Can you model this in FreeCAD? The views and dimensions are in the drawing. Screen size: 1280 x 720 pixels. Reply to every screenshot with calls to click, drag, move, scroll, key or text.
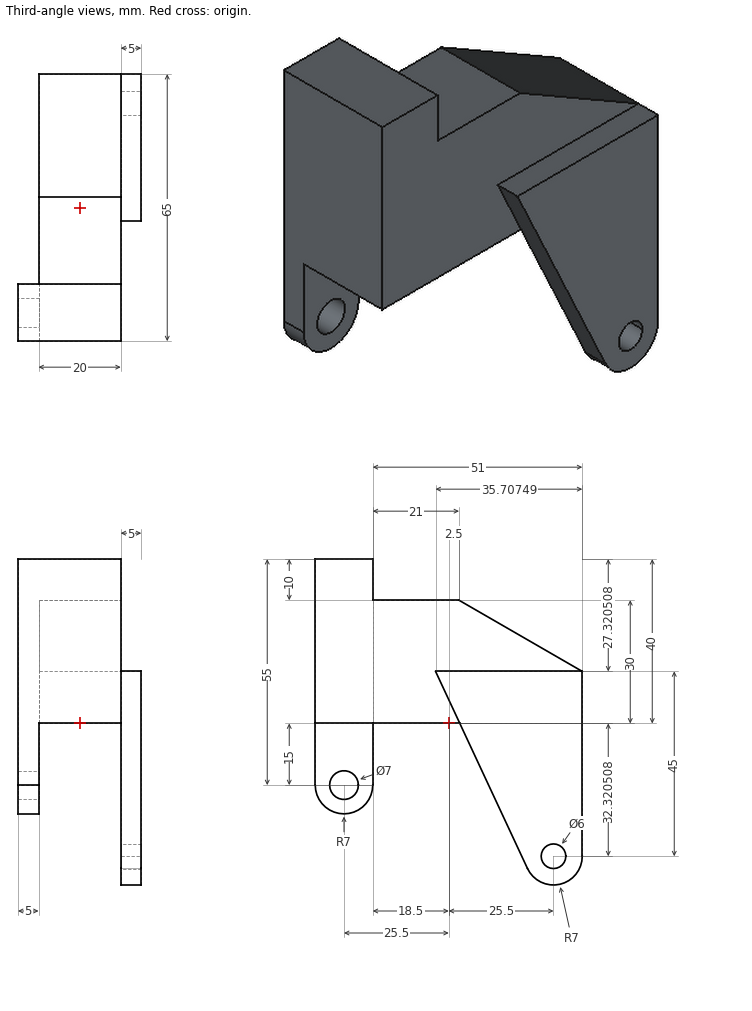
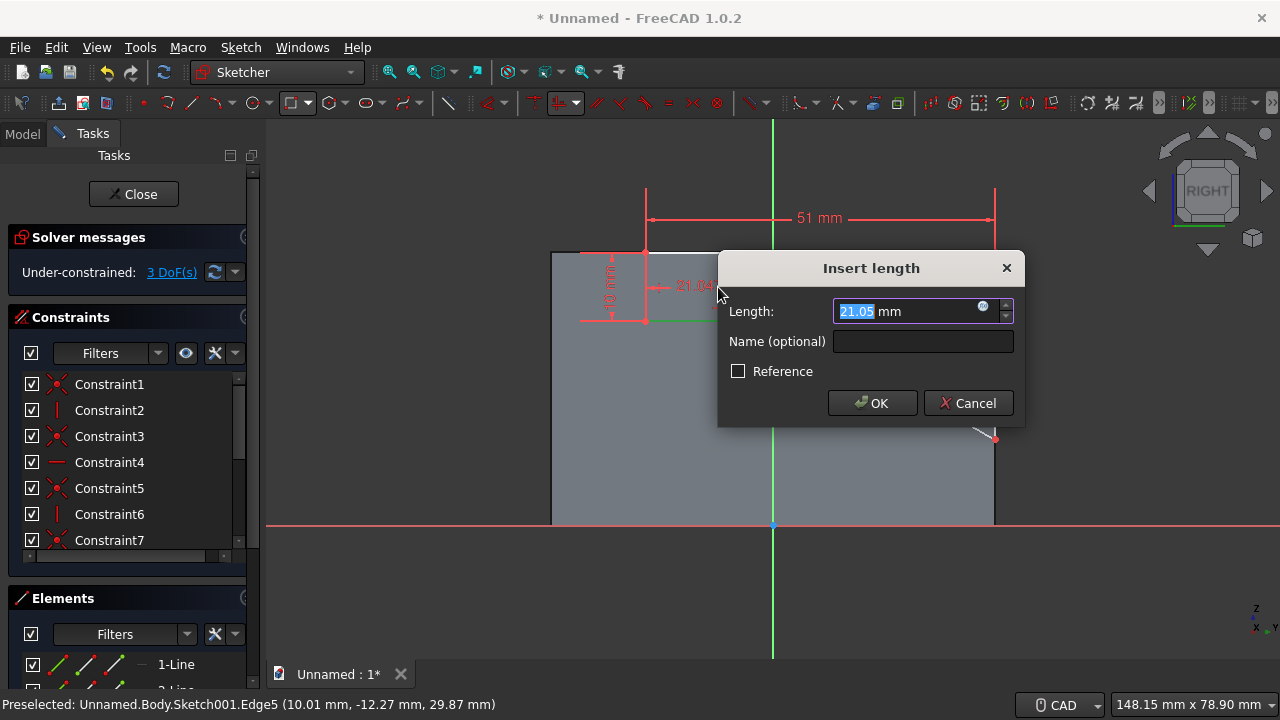
text(21)
key(Return)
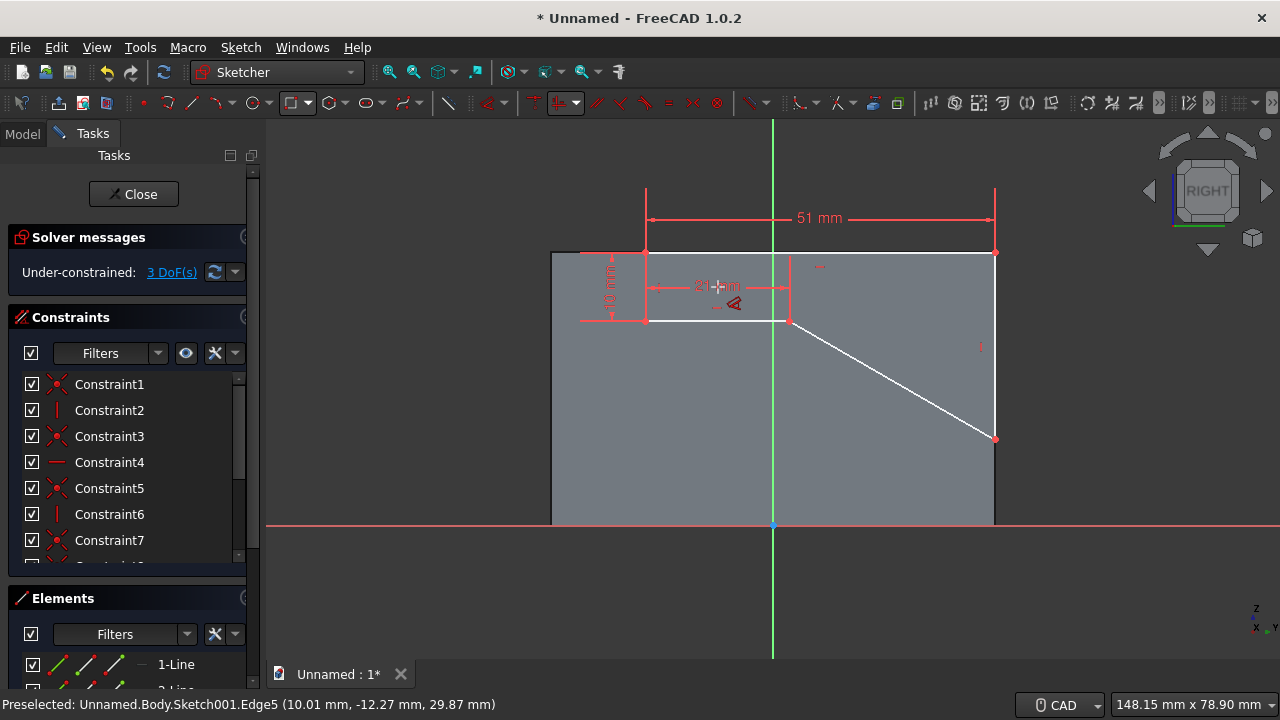
click(790, 321)
click(739, 424)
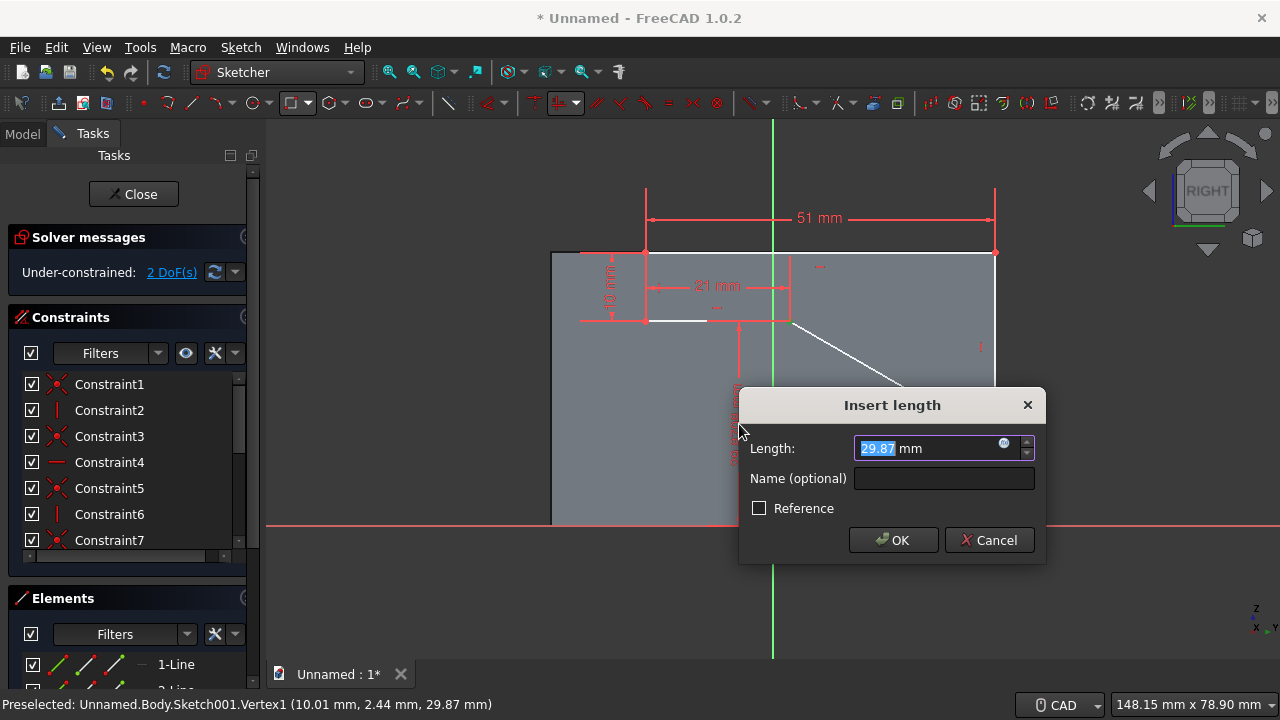
text(30)
key(Return)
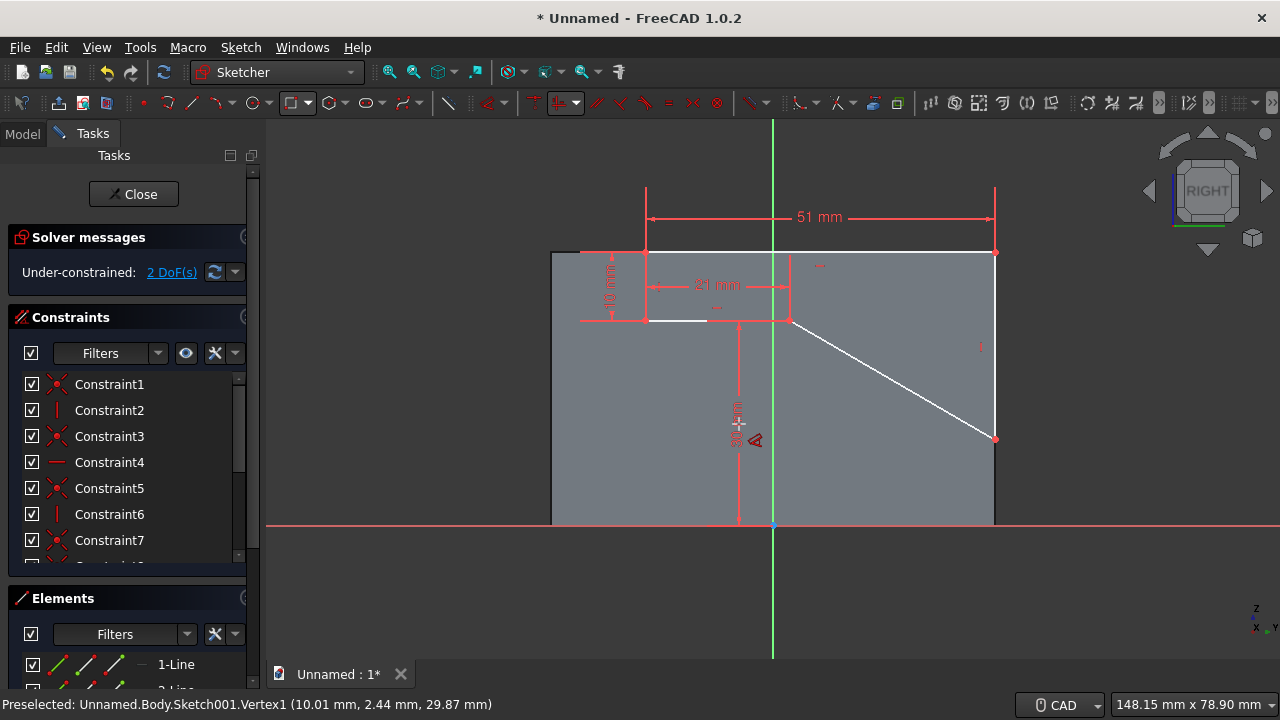
scroll(790, 321, up, 5)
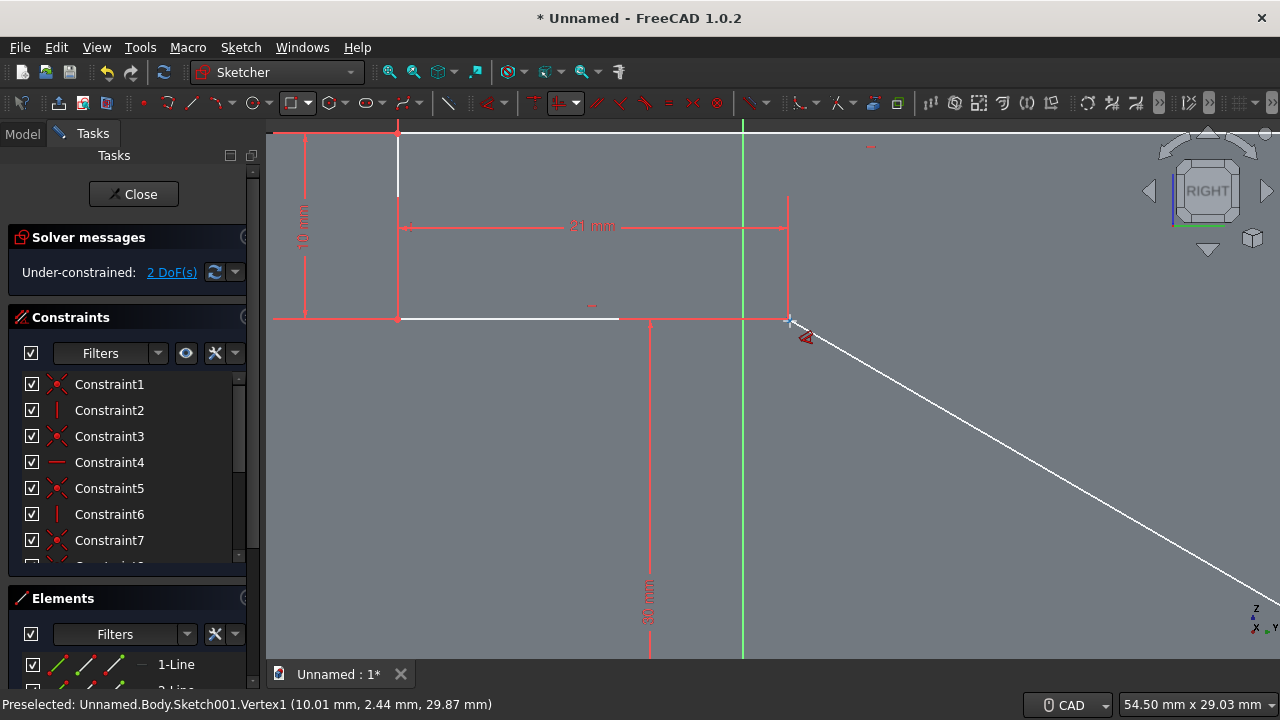
click(788, 319)
click(766, 285)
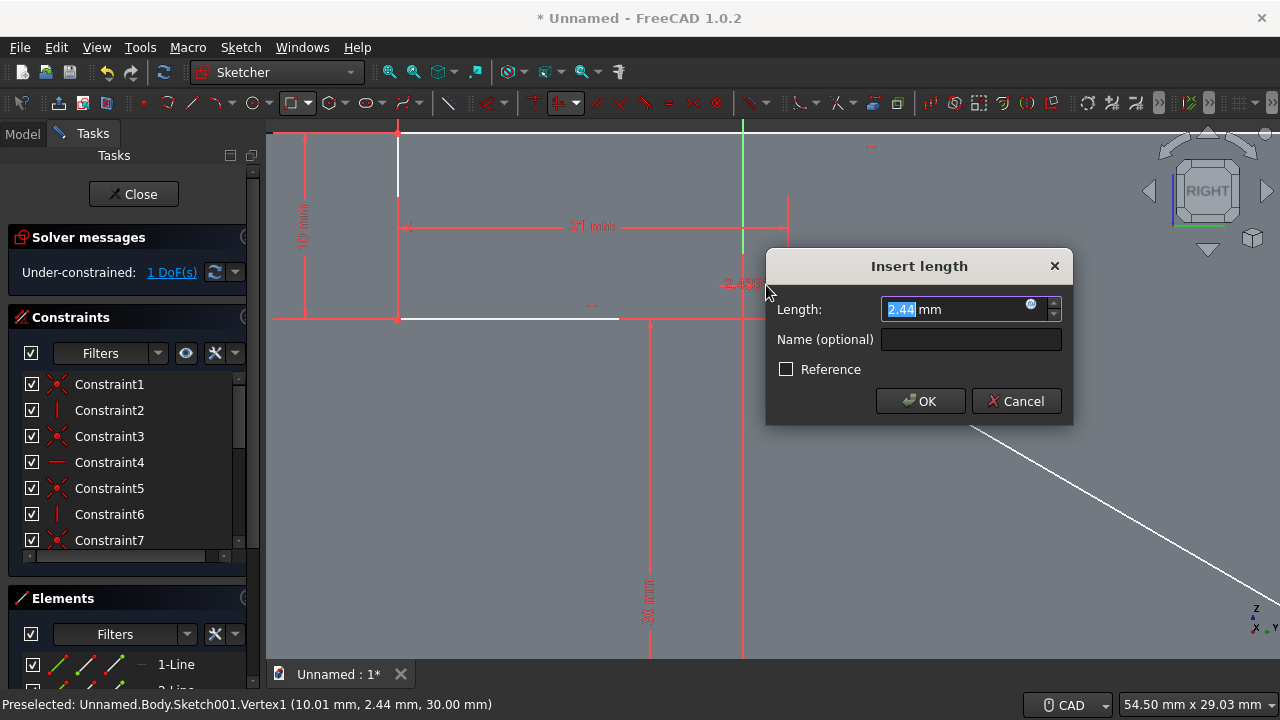
text(2.5)
key(Return)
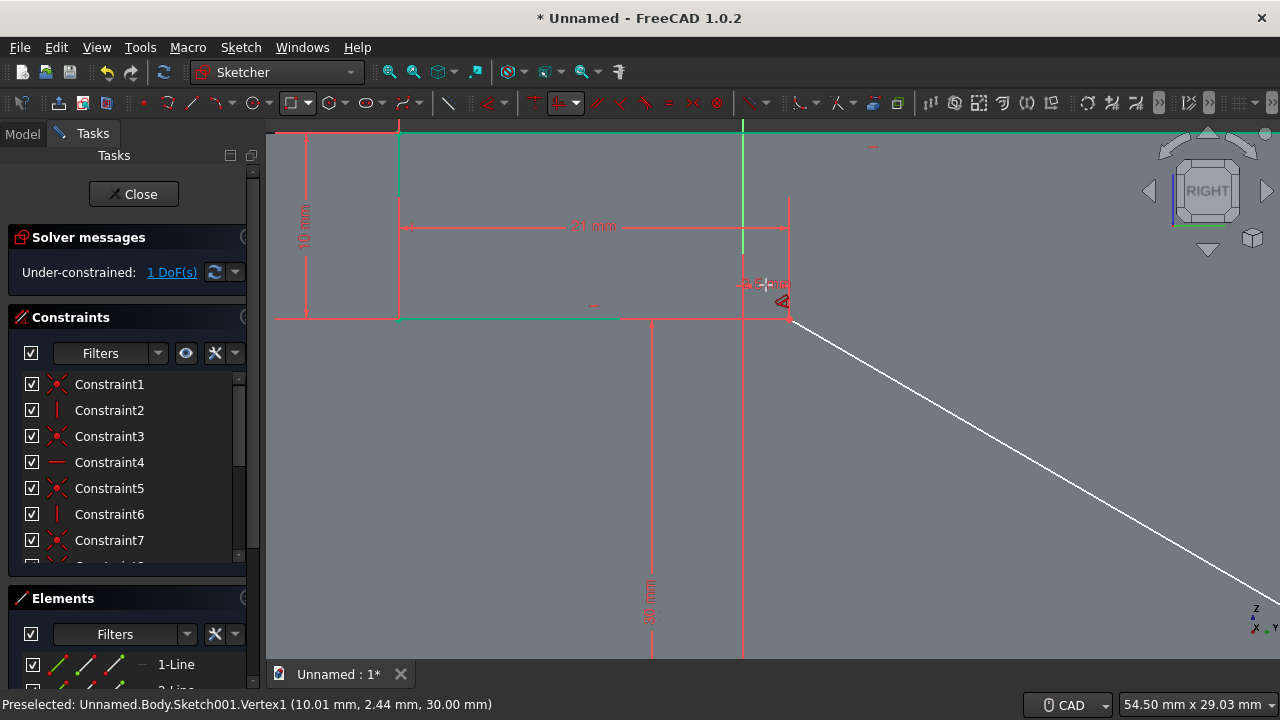
scroll(567, 294, down, 4)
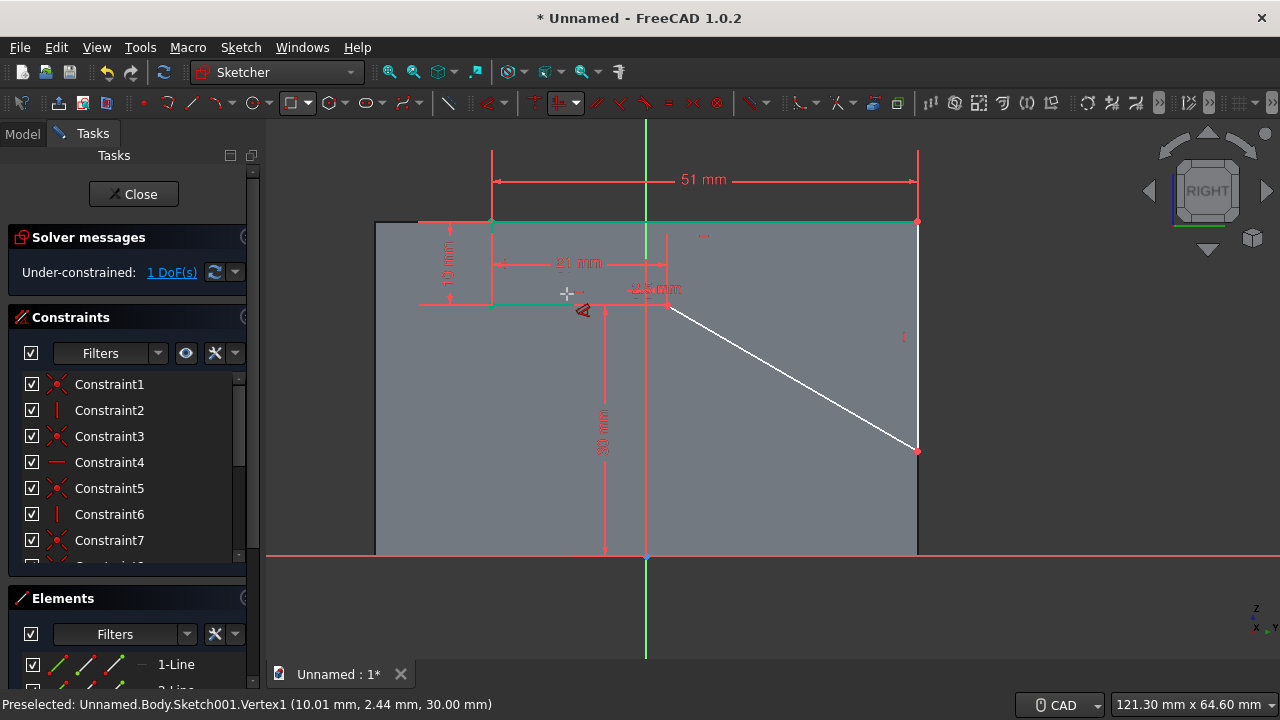
click(918, 383)
click(952, 337)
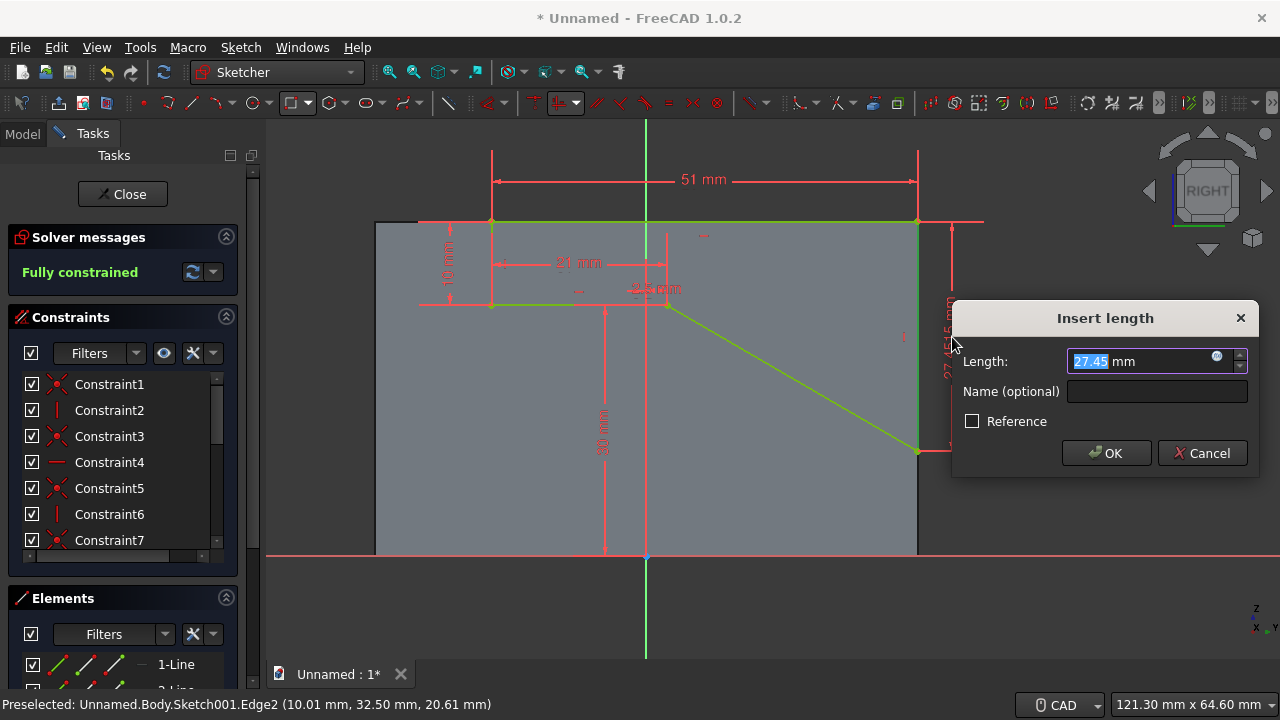
text(27.320508)
key(Return)
key(Escape)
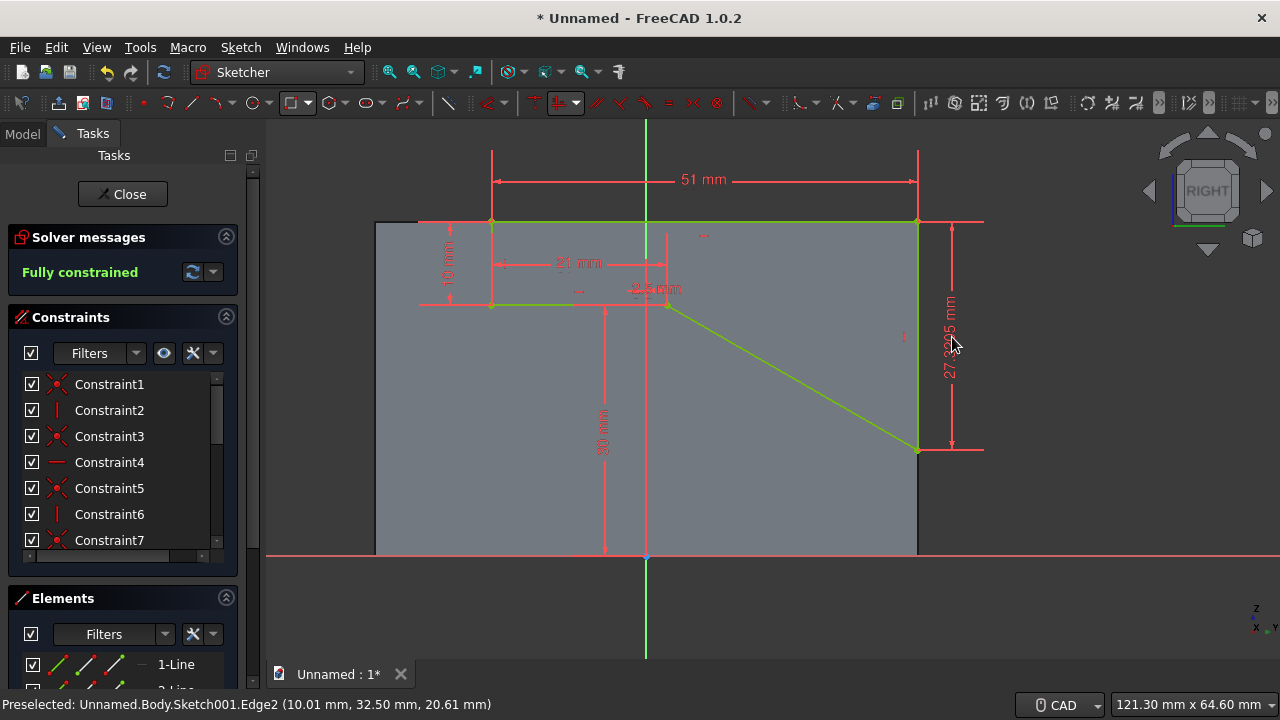
click(123, 194)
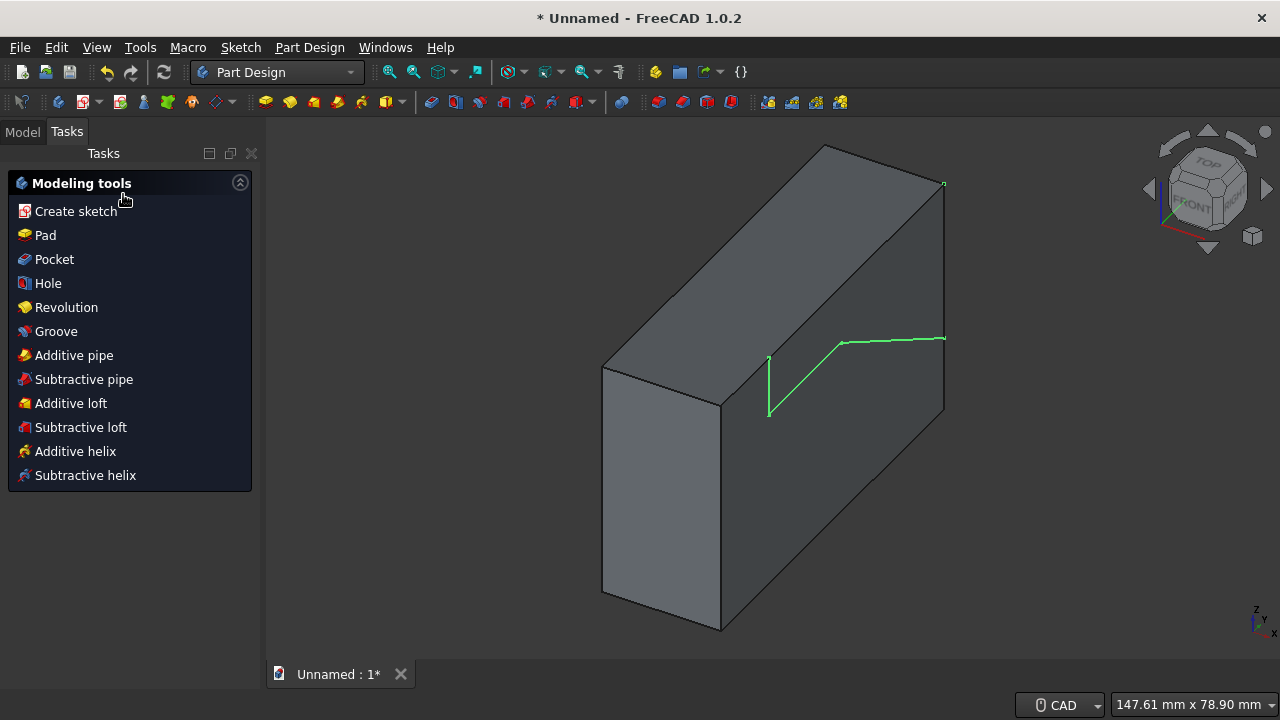
click(432, 102)